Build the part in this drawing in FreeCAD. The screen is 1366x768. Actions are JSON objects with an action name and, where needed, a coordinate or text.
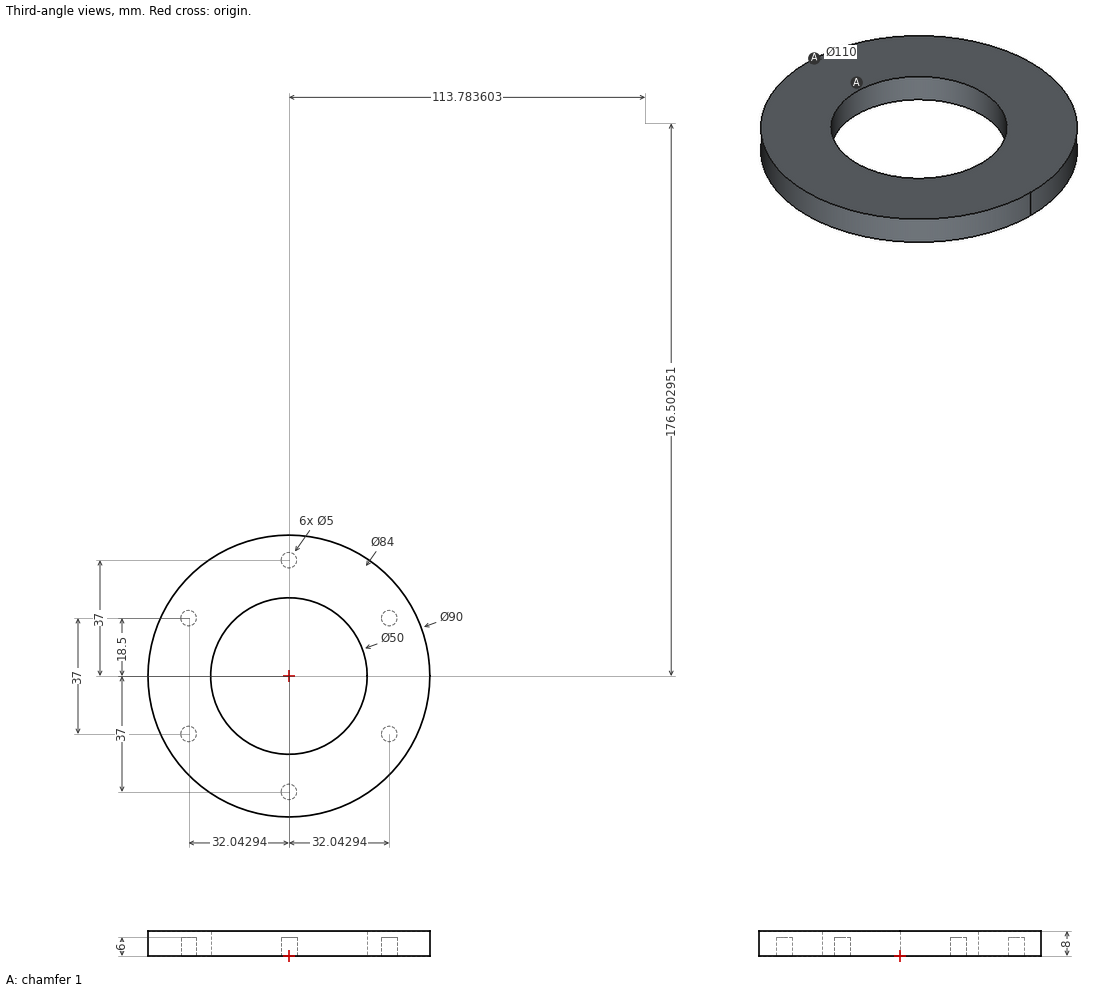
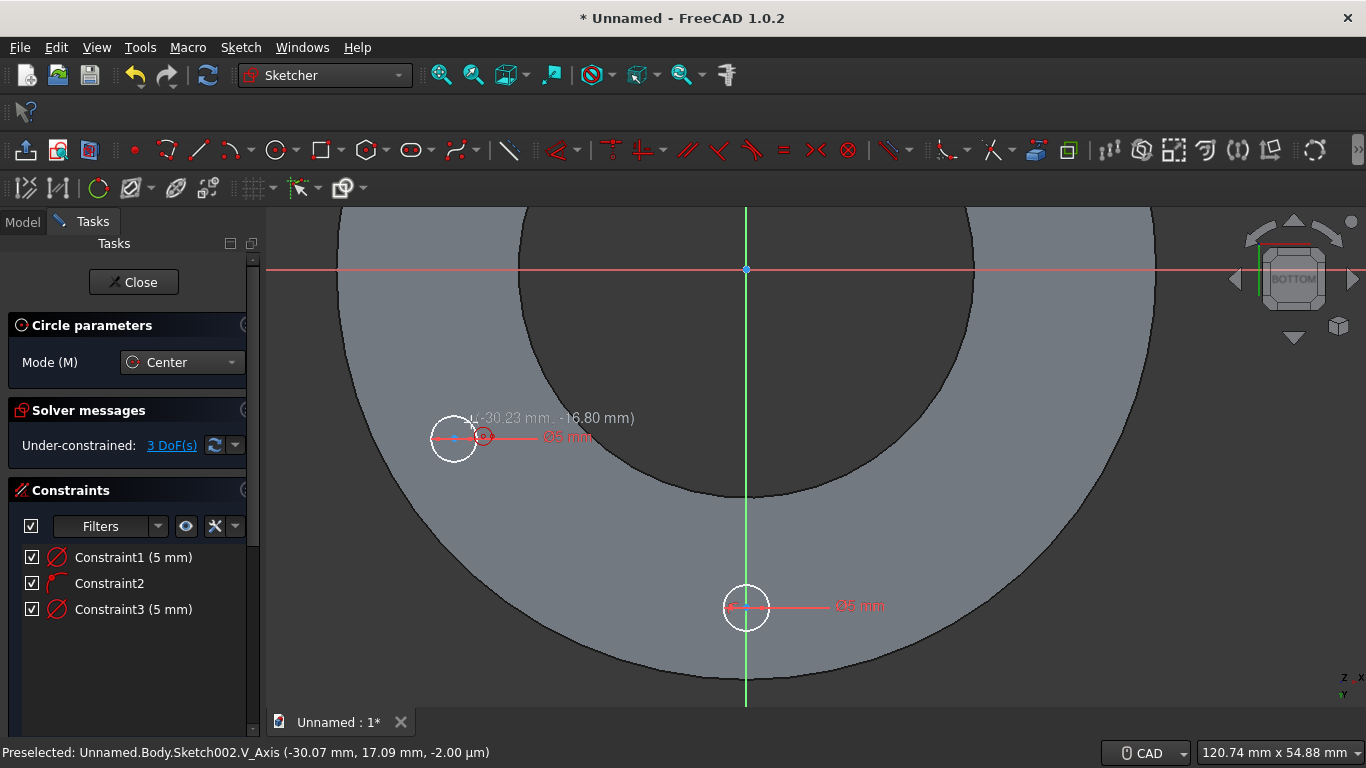
{"action": "scroll", "coordinate": [748, 610], "scroll_direction": "down", "scroll_amount": 4}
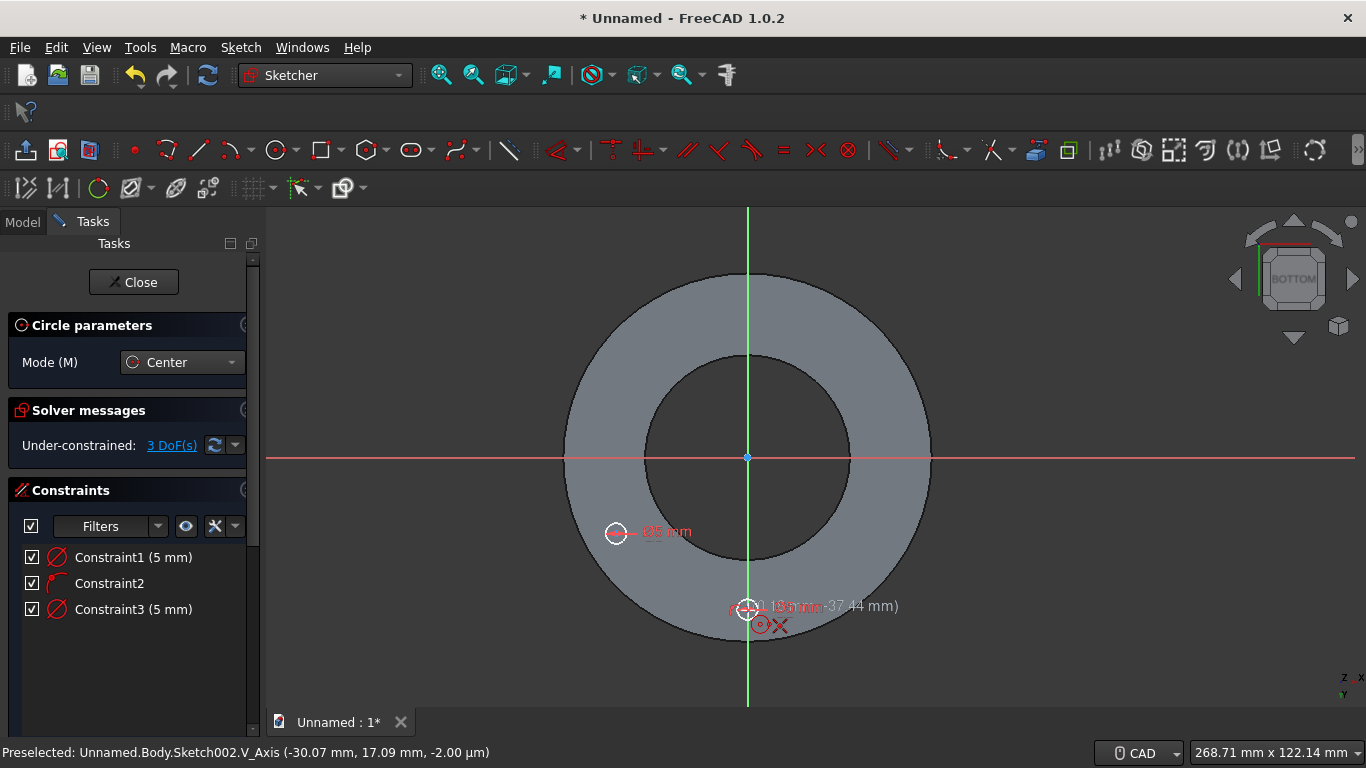
{"action": "scroll", "coordinate": [616, 382], "scroll_direction": "up", "scroll_amount": 4}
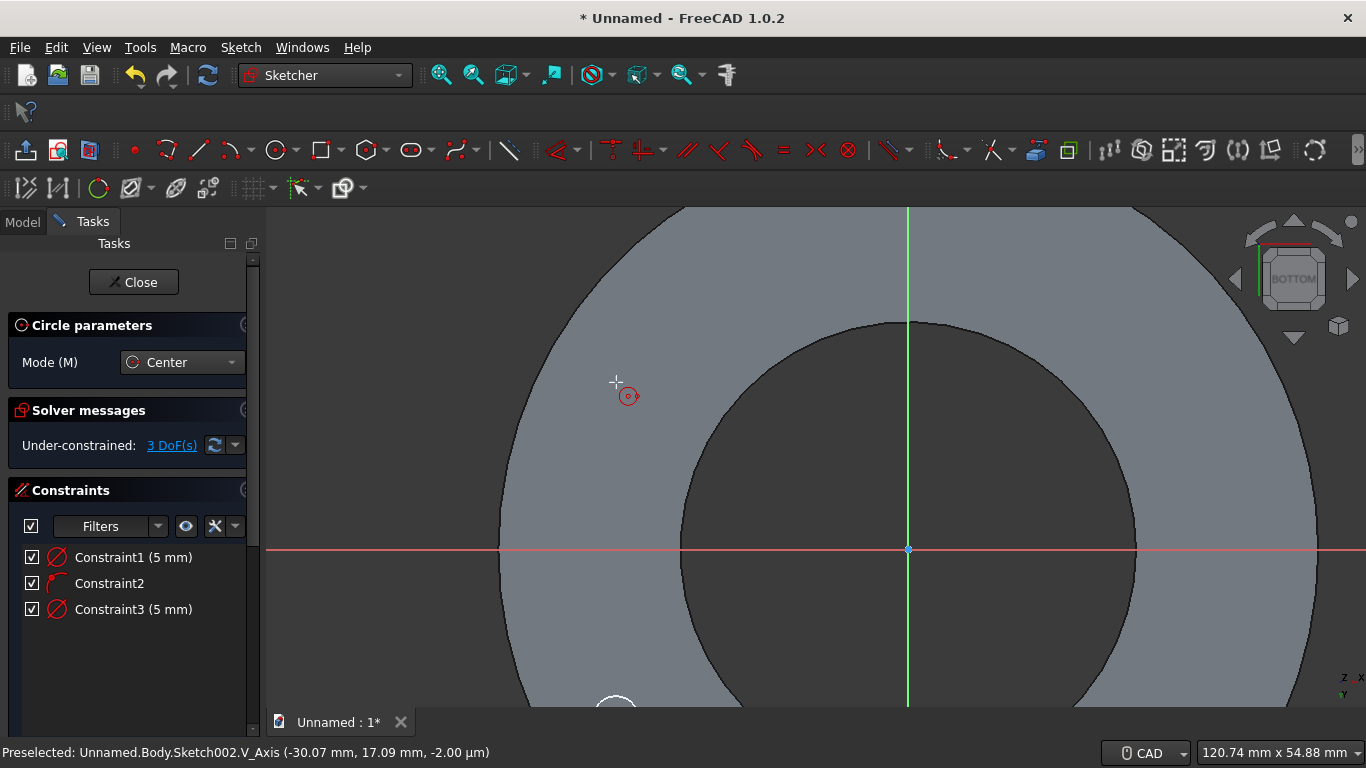
{"action": "left_click", "coordinate": [616, 381]}
{"action": "mouse_move", "coordinate": [632, 365]}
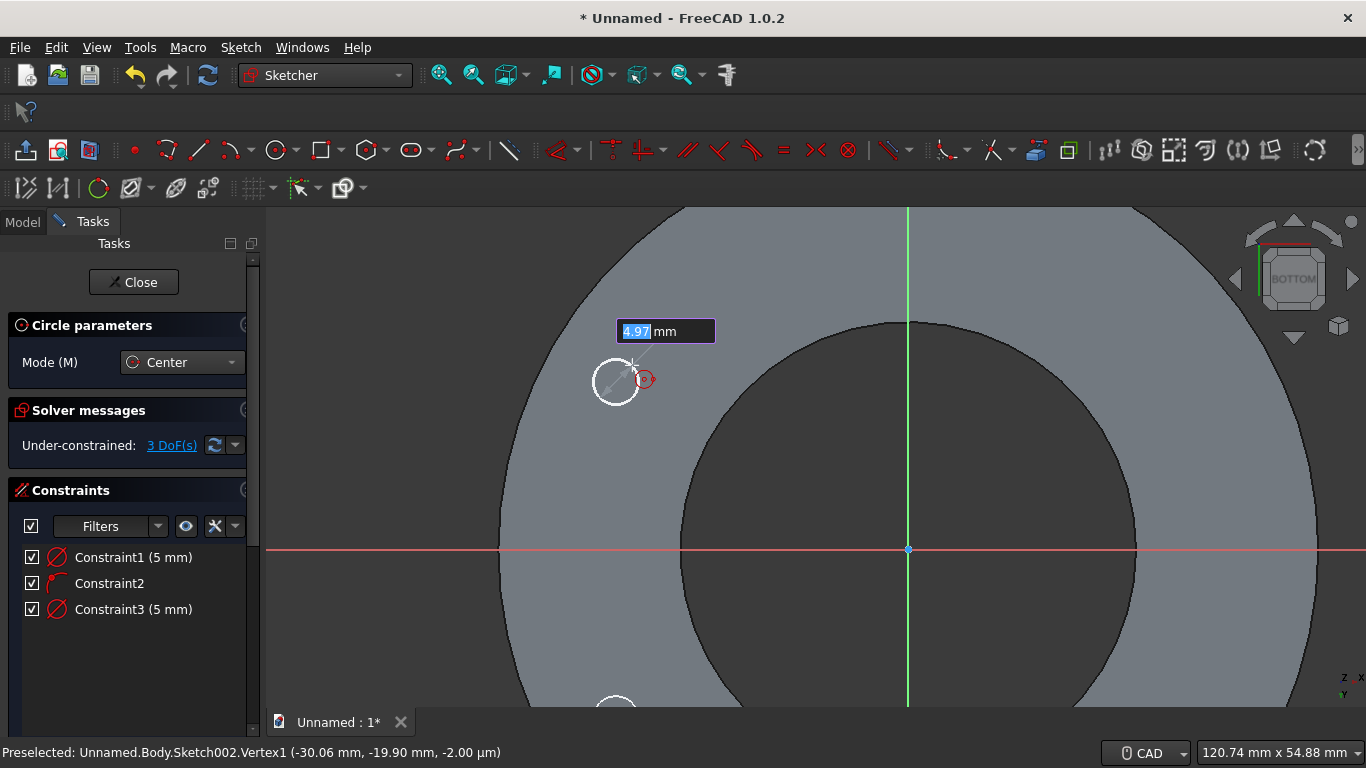
{"action": "type", "text": "5"}
{"action": "key", "text": "Return"}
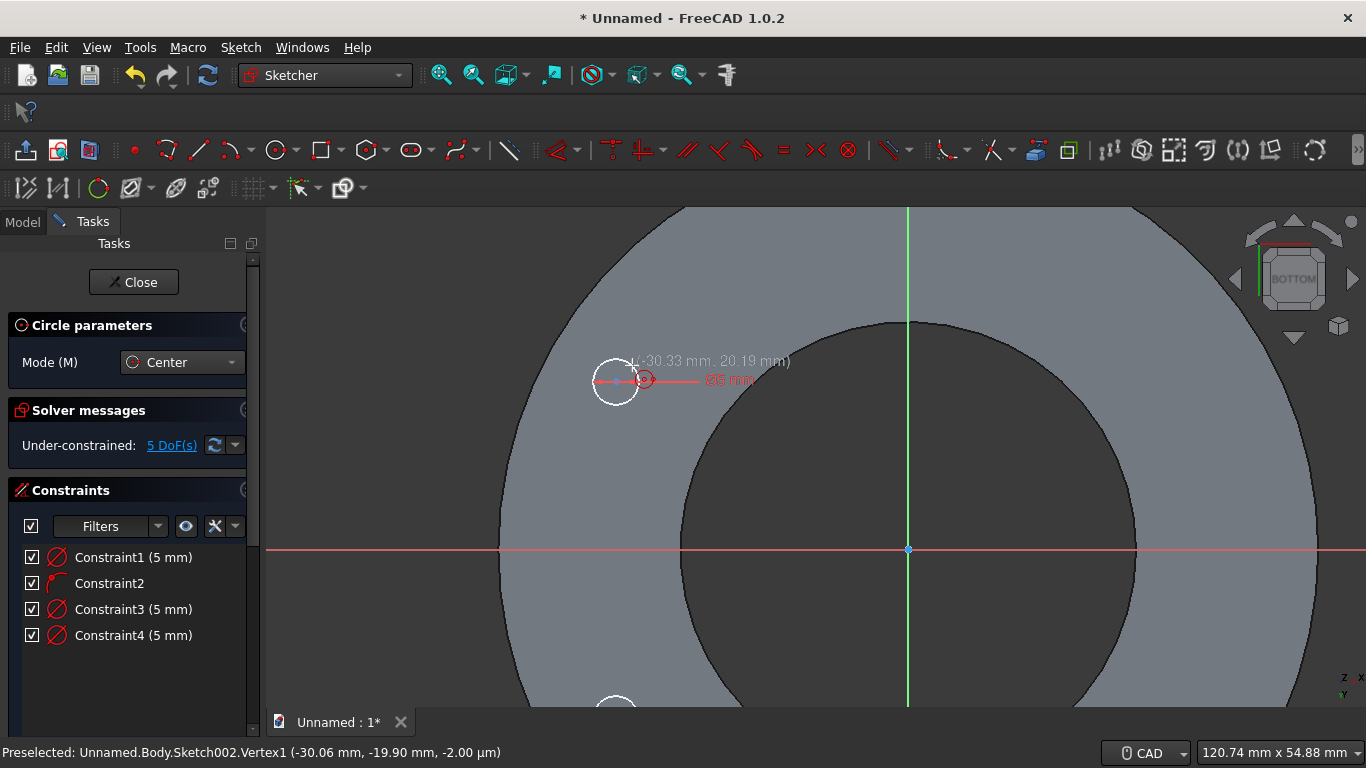
{"action": "scroll", "coordinate": [616, 381], "scroll_direction": "down", "scroll_amount": 4}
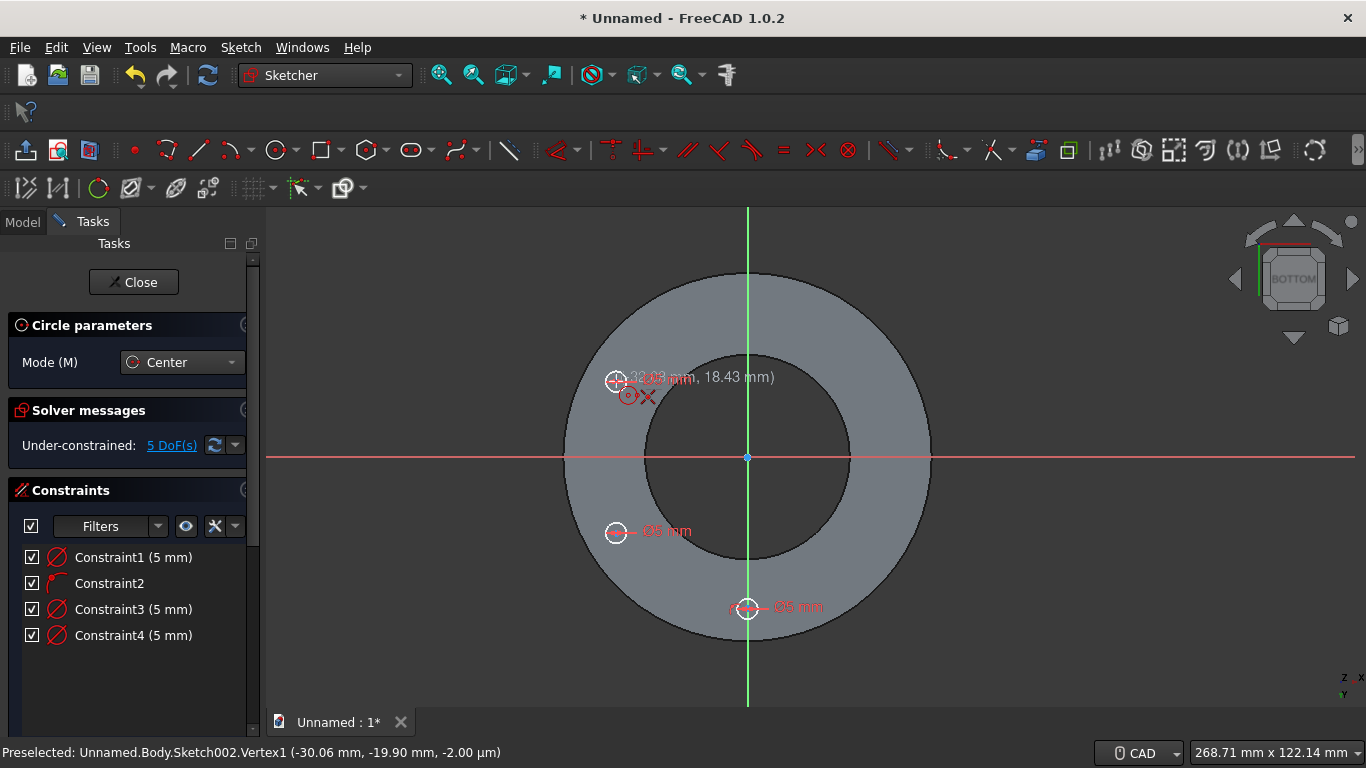
{"action": "scroll", "coordinate": [748, 306], "scroll_direction": "up", "scroll_amount": 4}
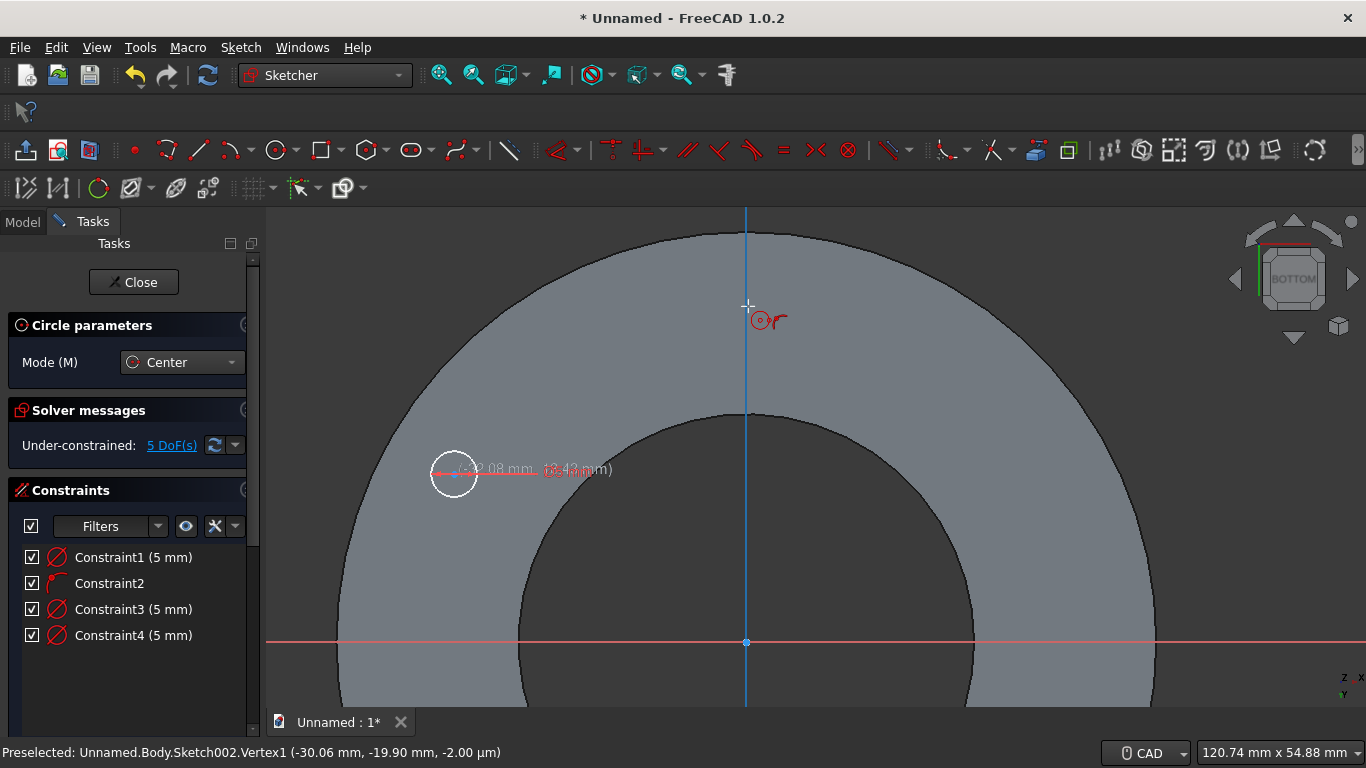
{"action": "left_click", "coordinate": [746, 305]}
{"action": "mouse_move", "coordinate": [762, 289]}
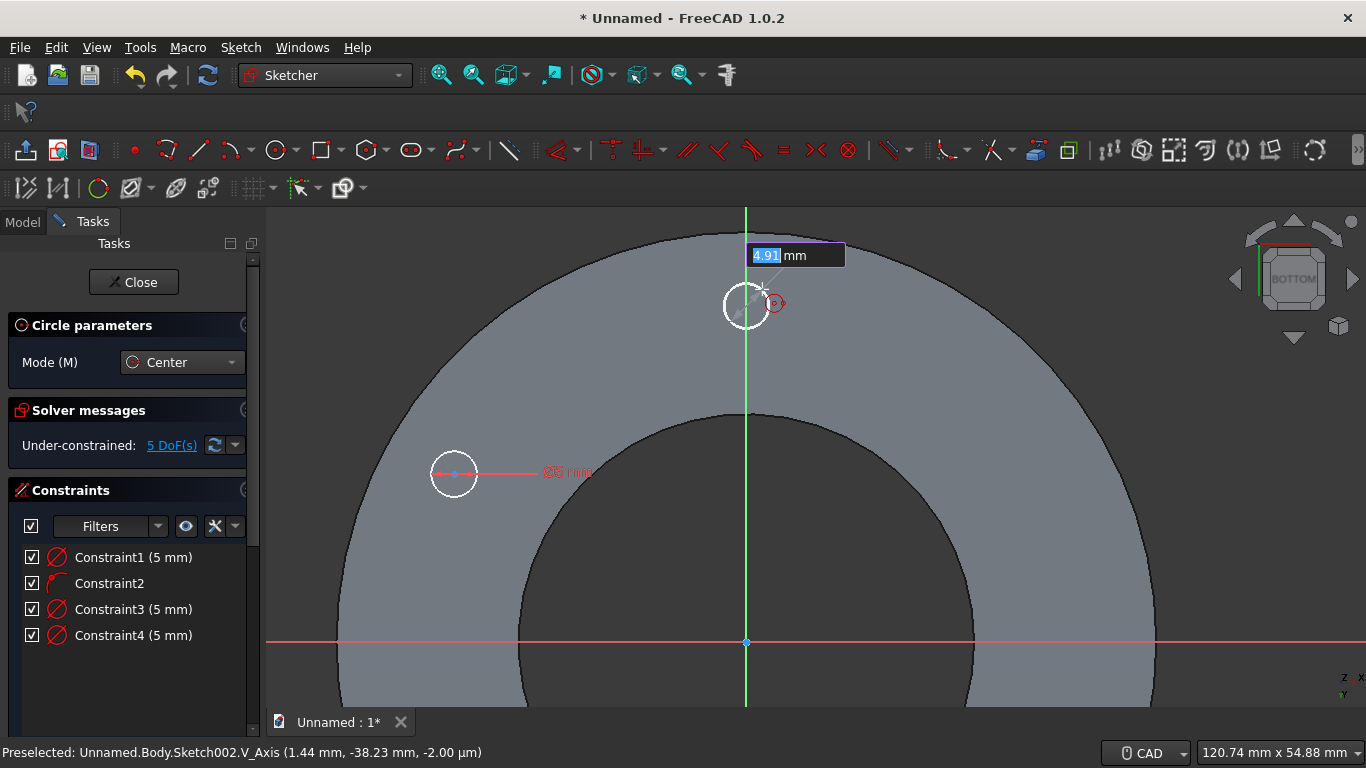
{"action": "type", "text": "5"}
{"action": "key", "text": "Return"}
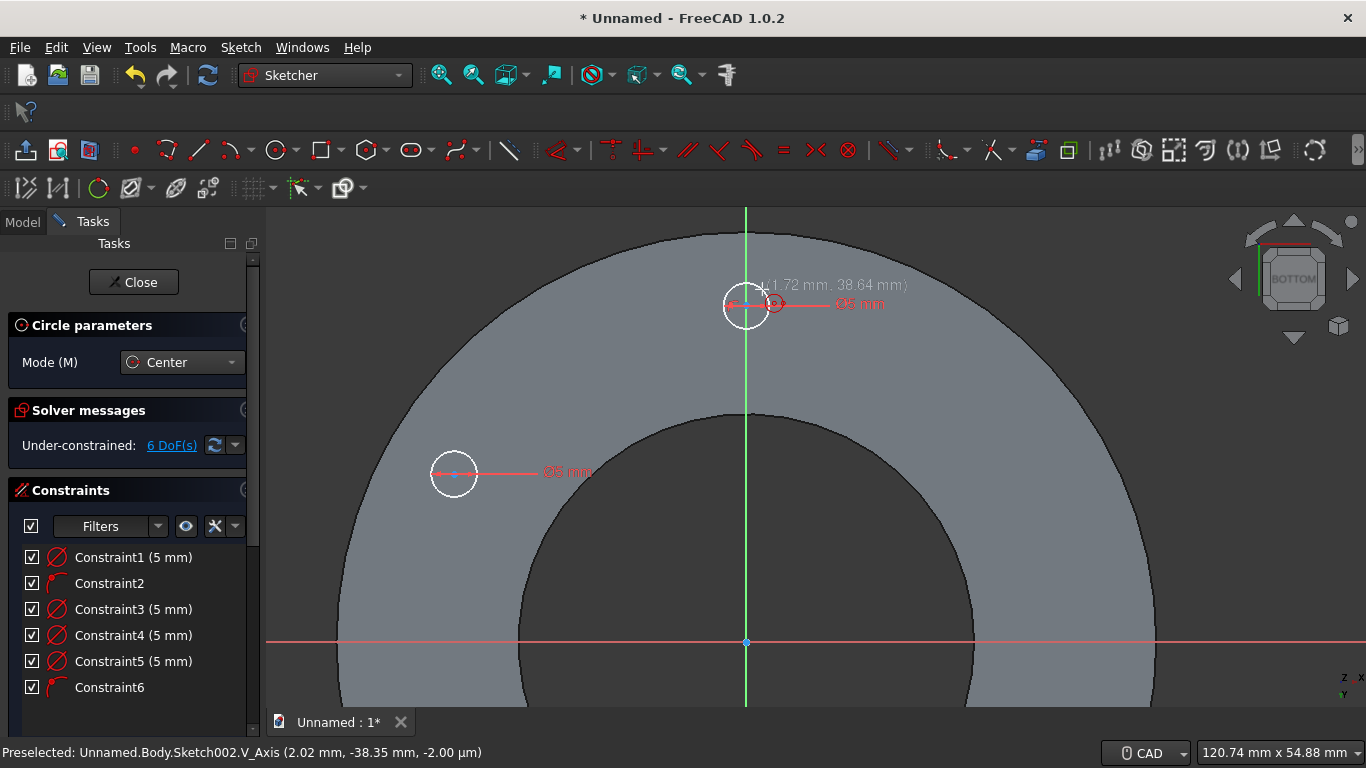
{"action": "left_click", "coordinate": [1038, 473]}
{"action": "mouse_move", "coordinate": [1054, 457]}